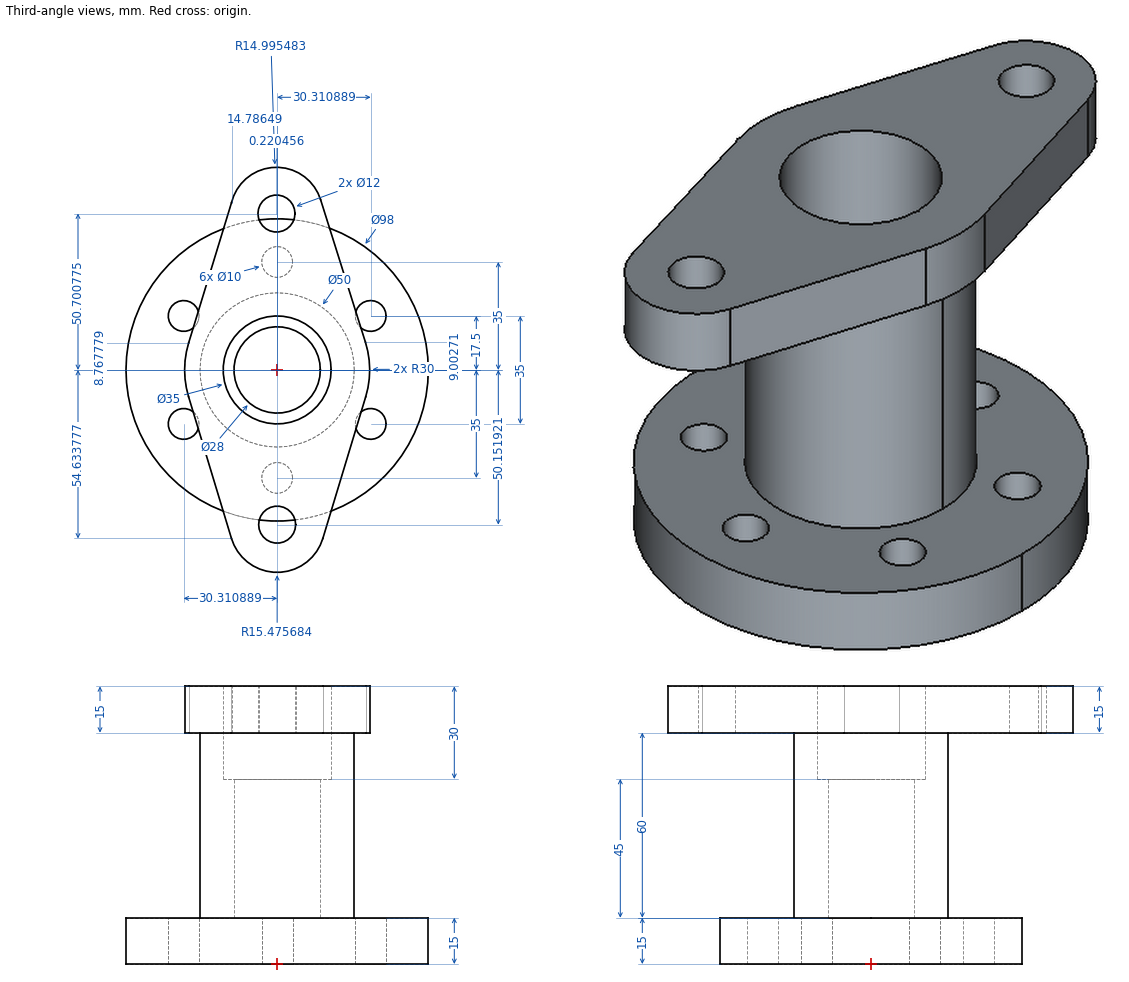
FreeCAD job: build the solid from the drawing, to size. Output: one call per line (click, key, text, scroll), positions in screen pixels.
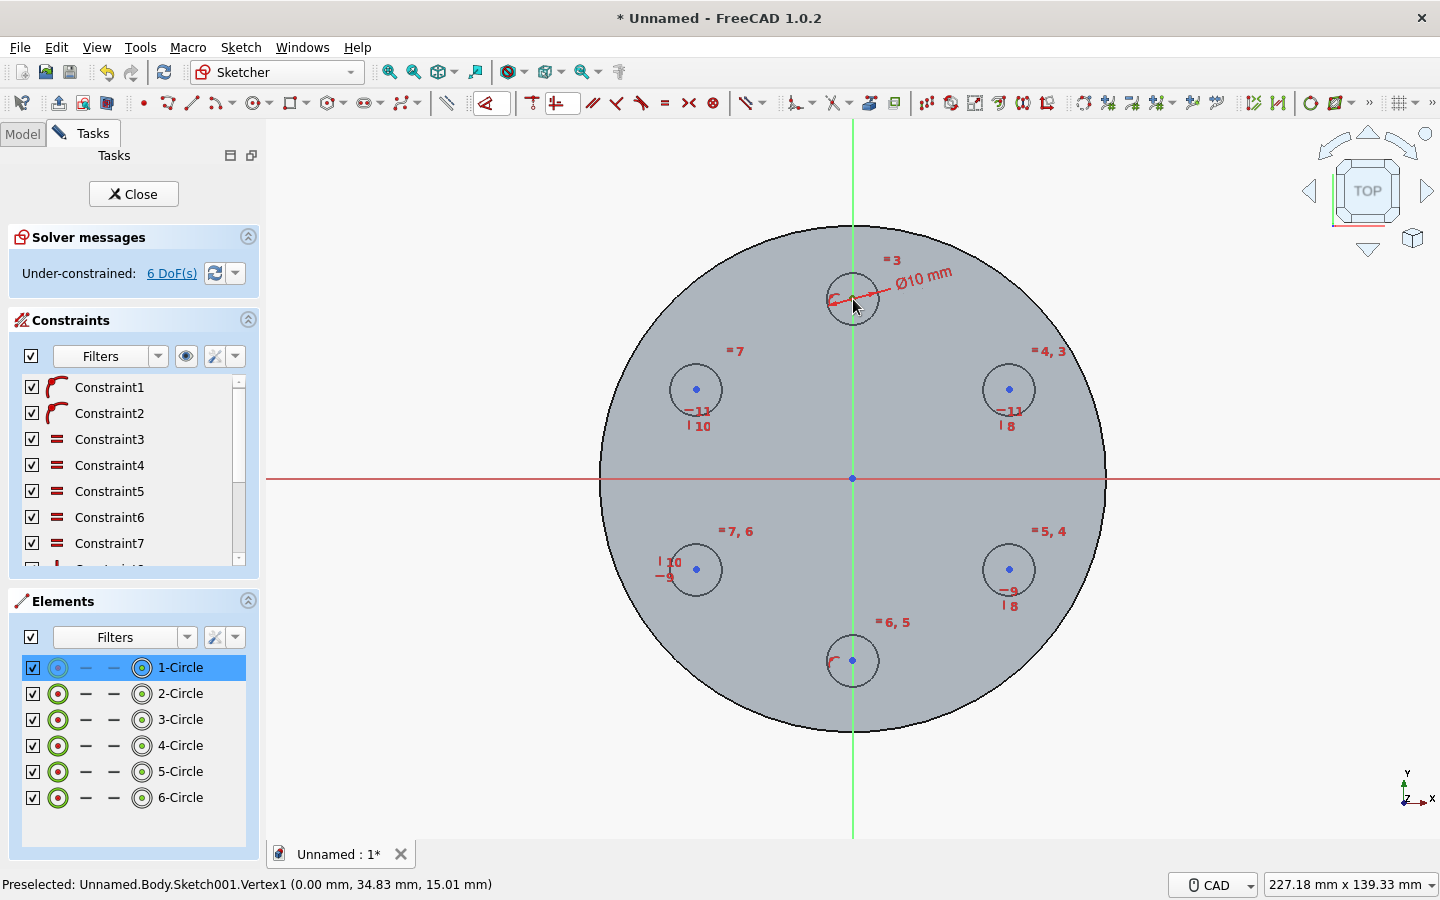
key(i)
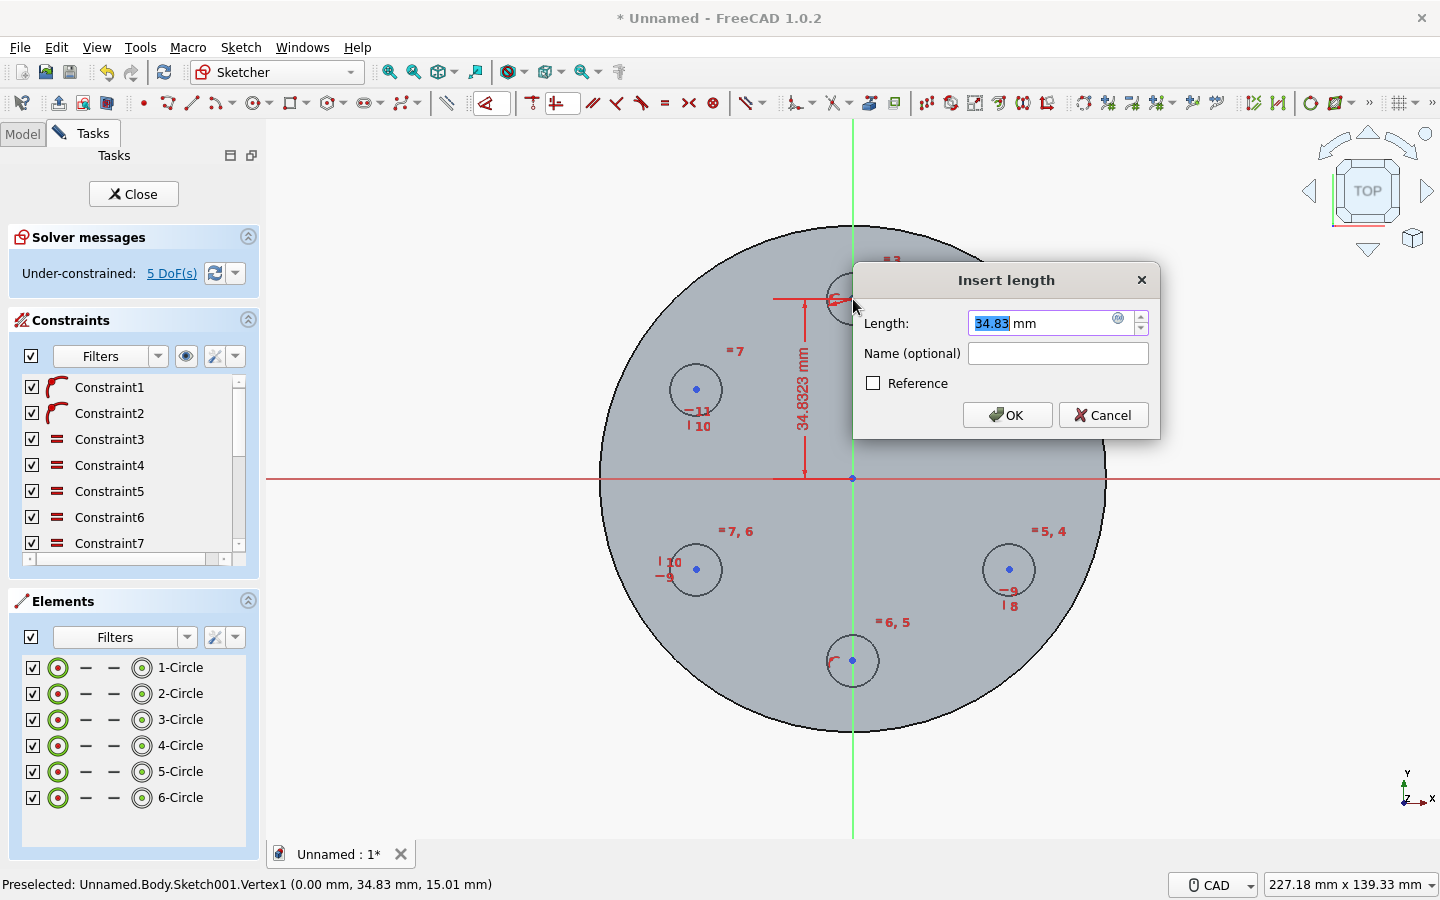
text(35)
key(Return)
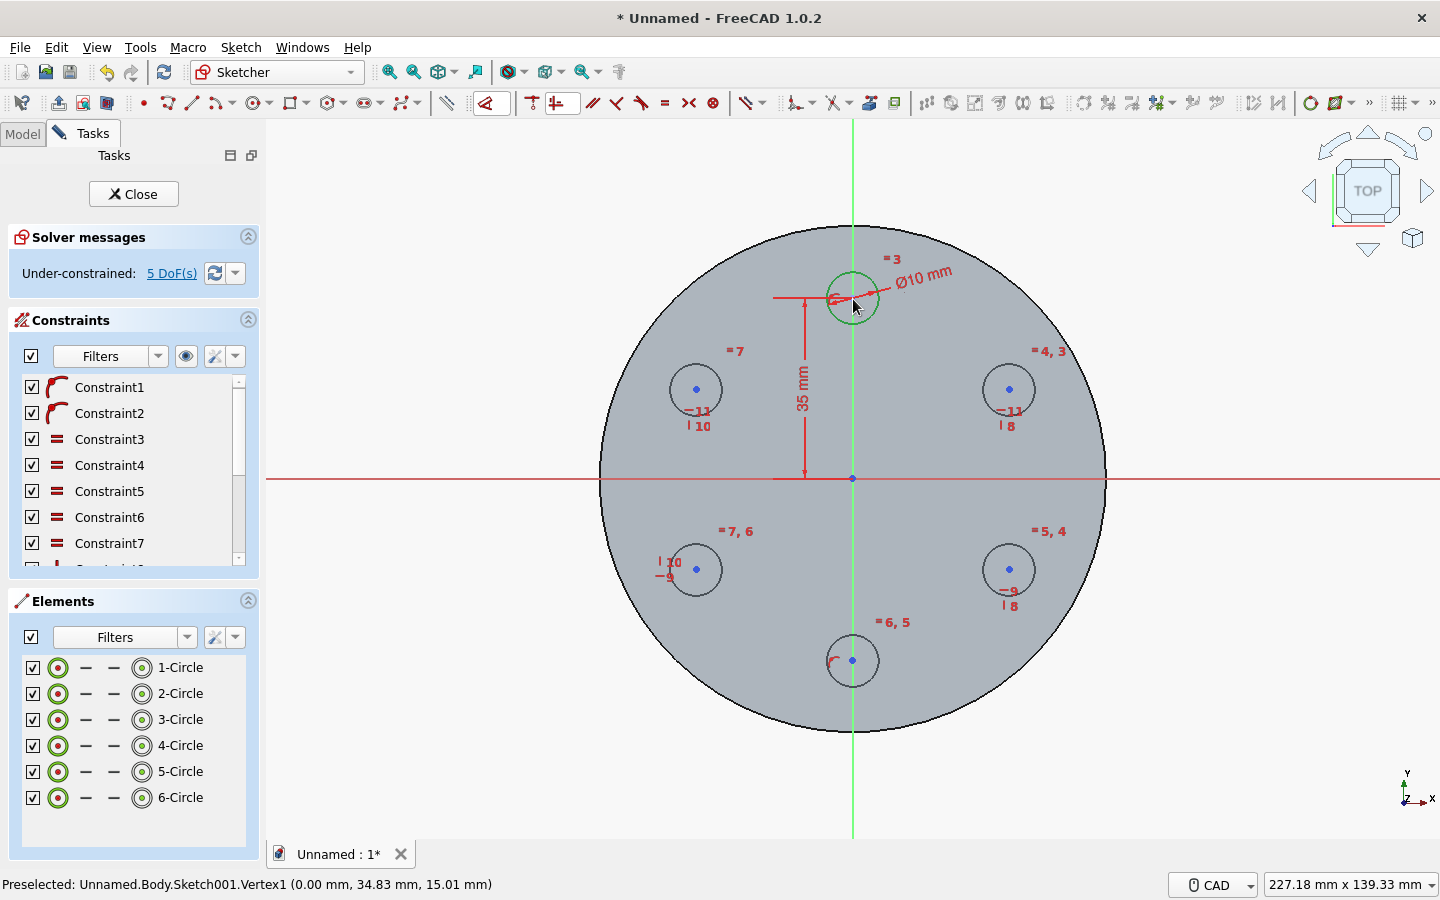
click(853, 661)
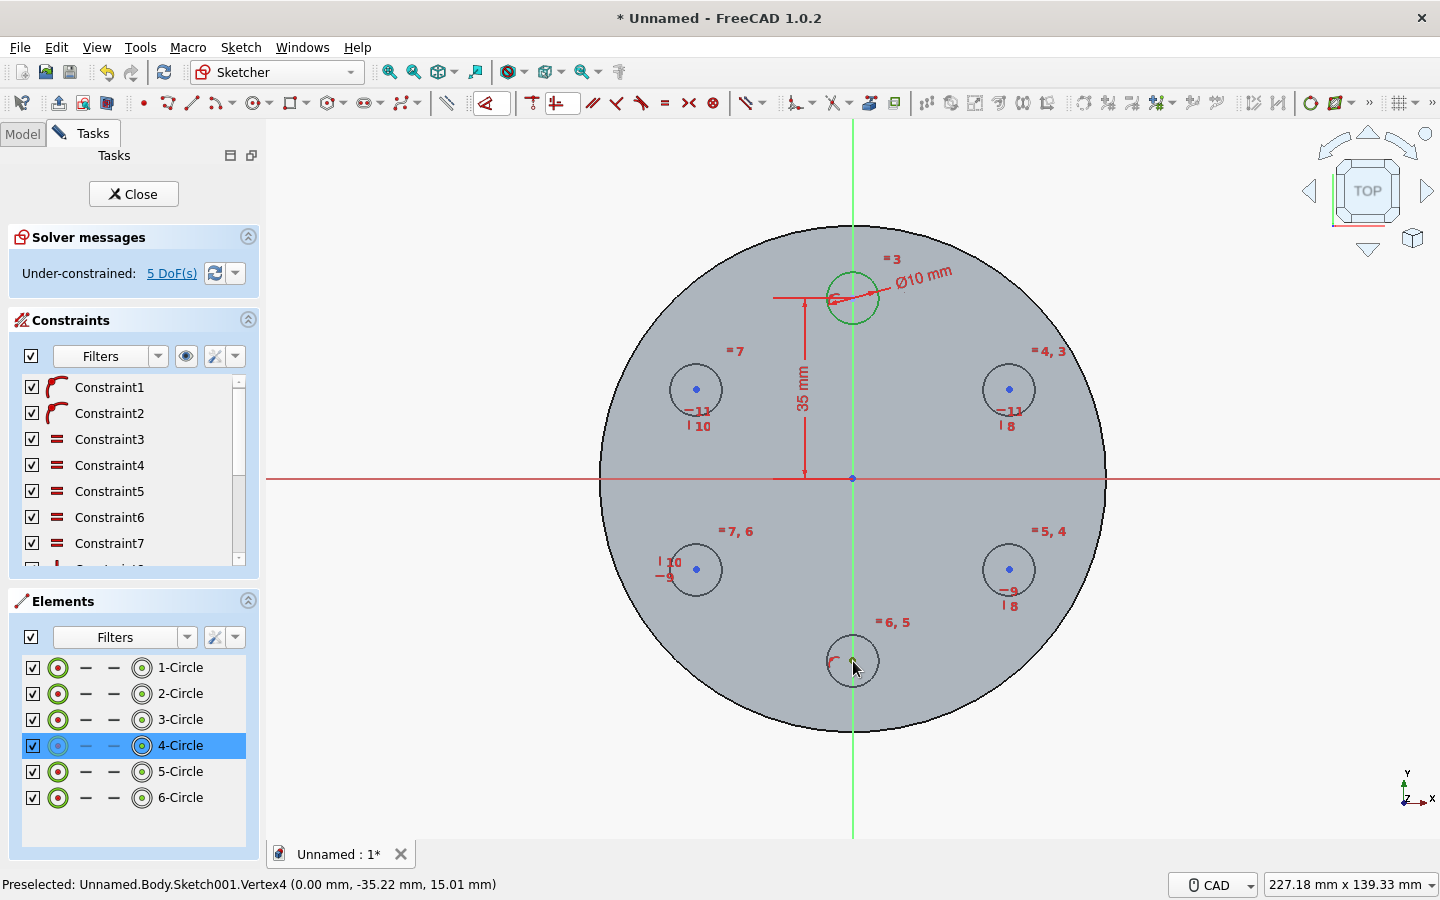
key(i)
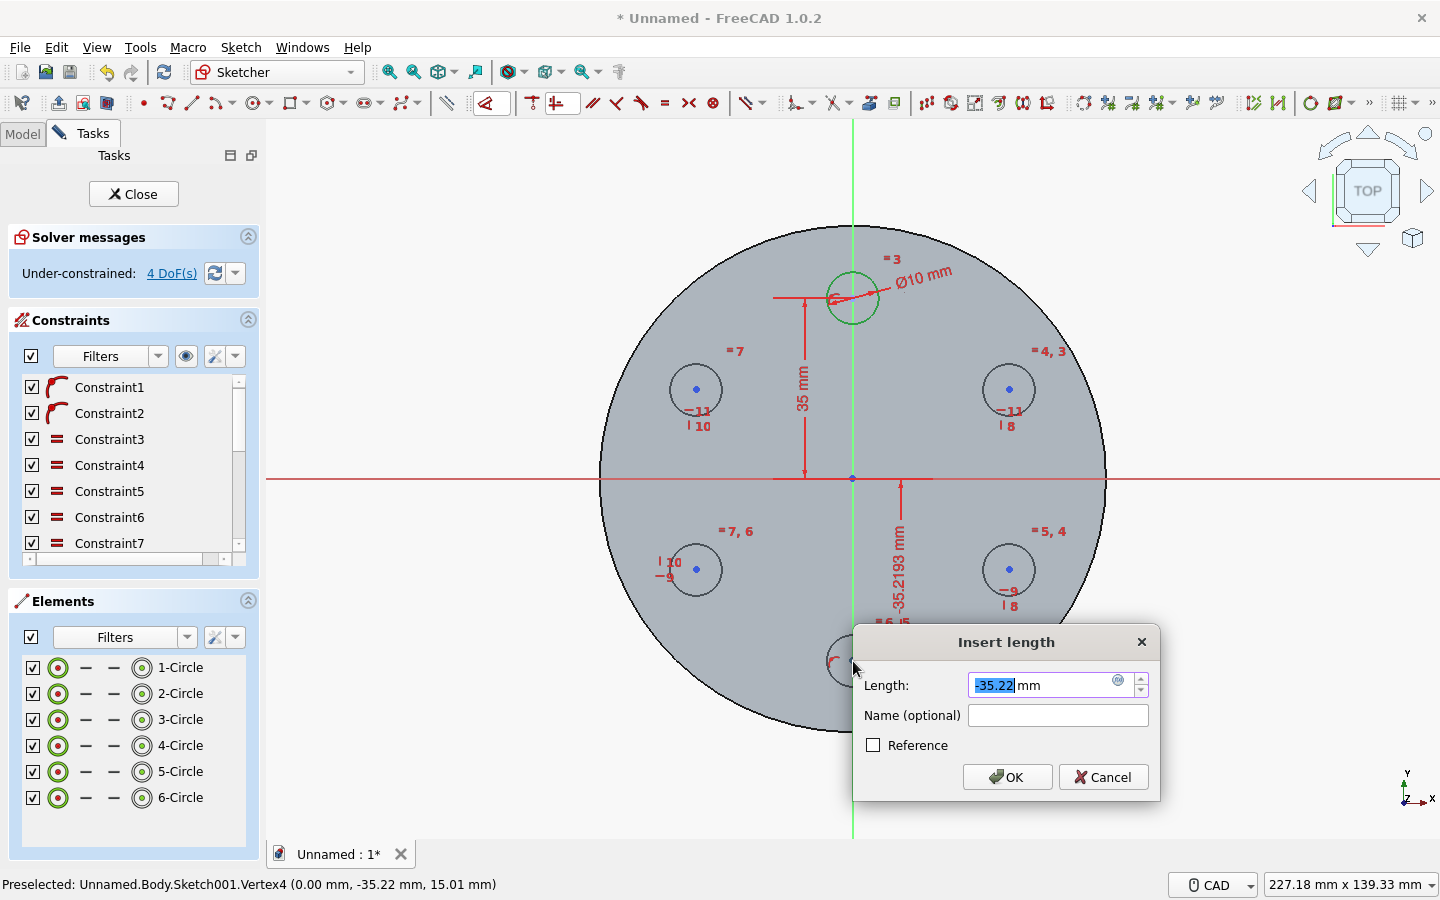
text(-35)
key(Return)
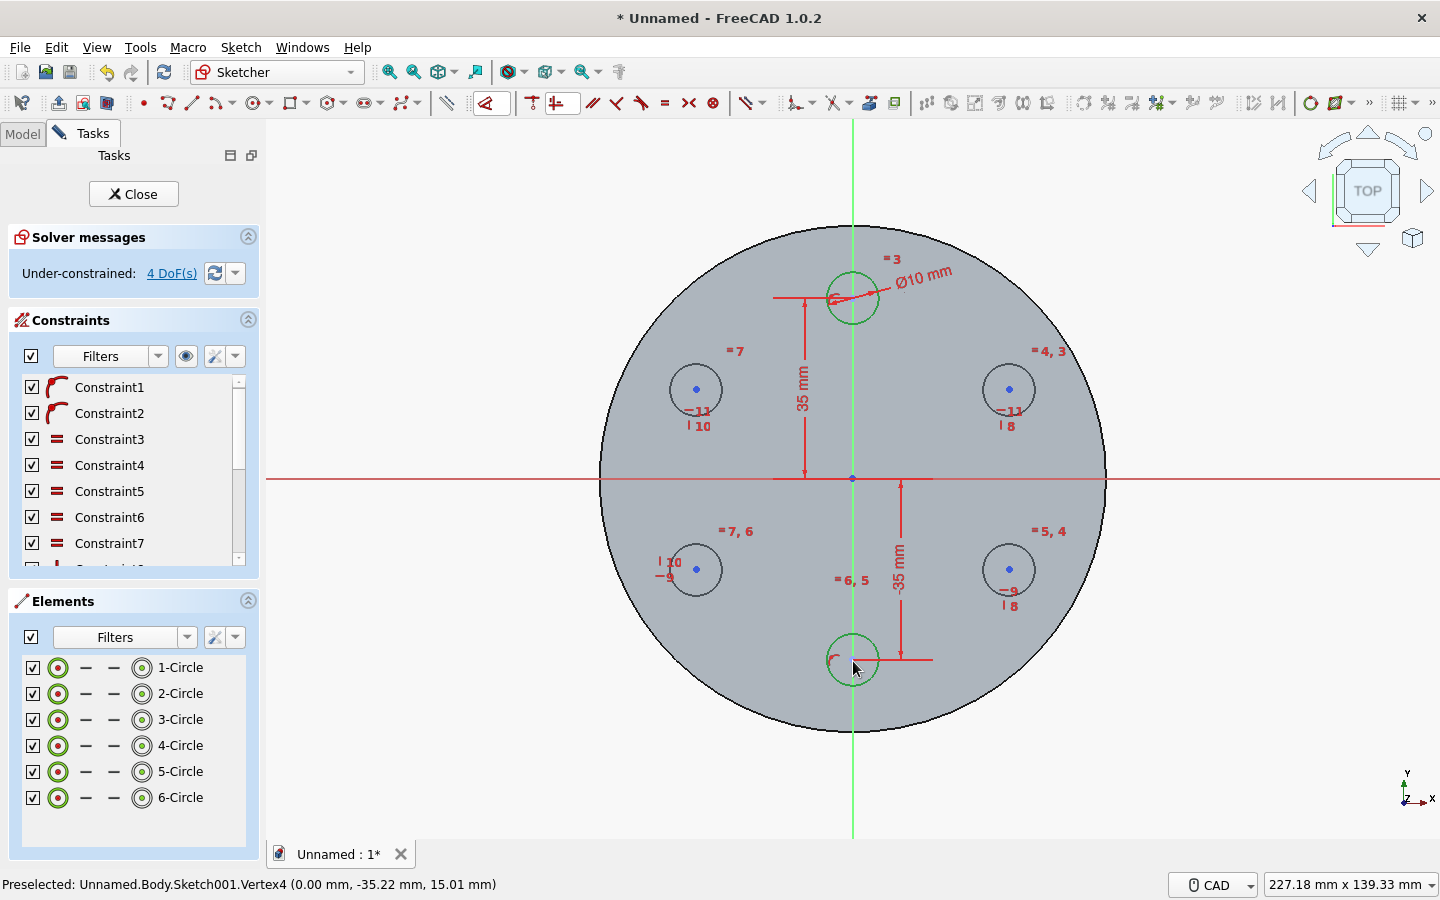
click(1009, 390)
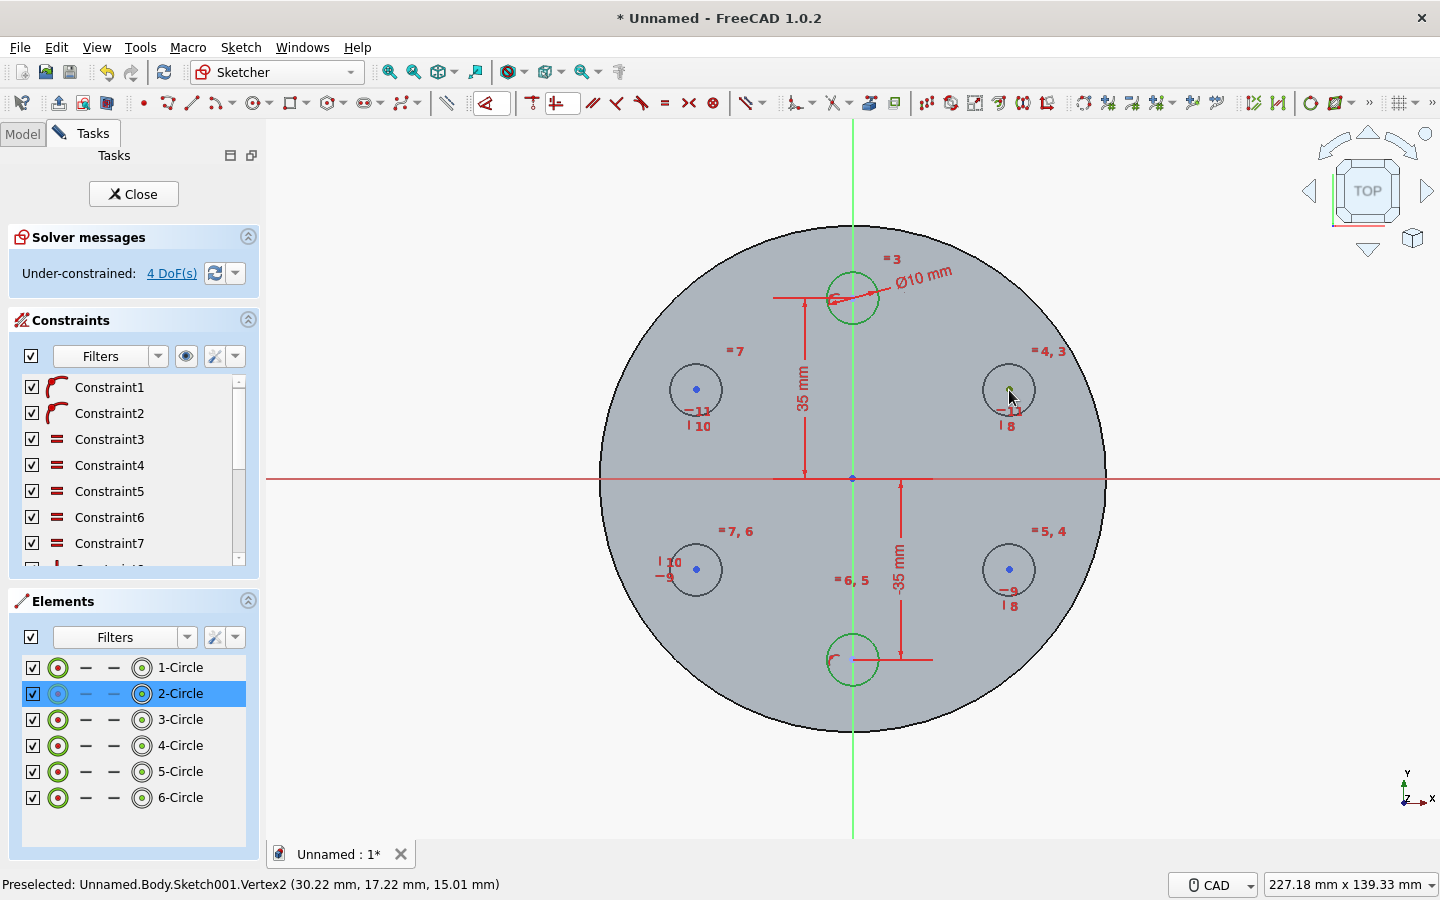
click(1009, 570)